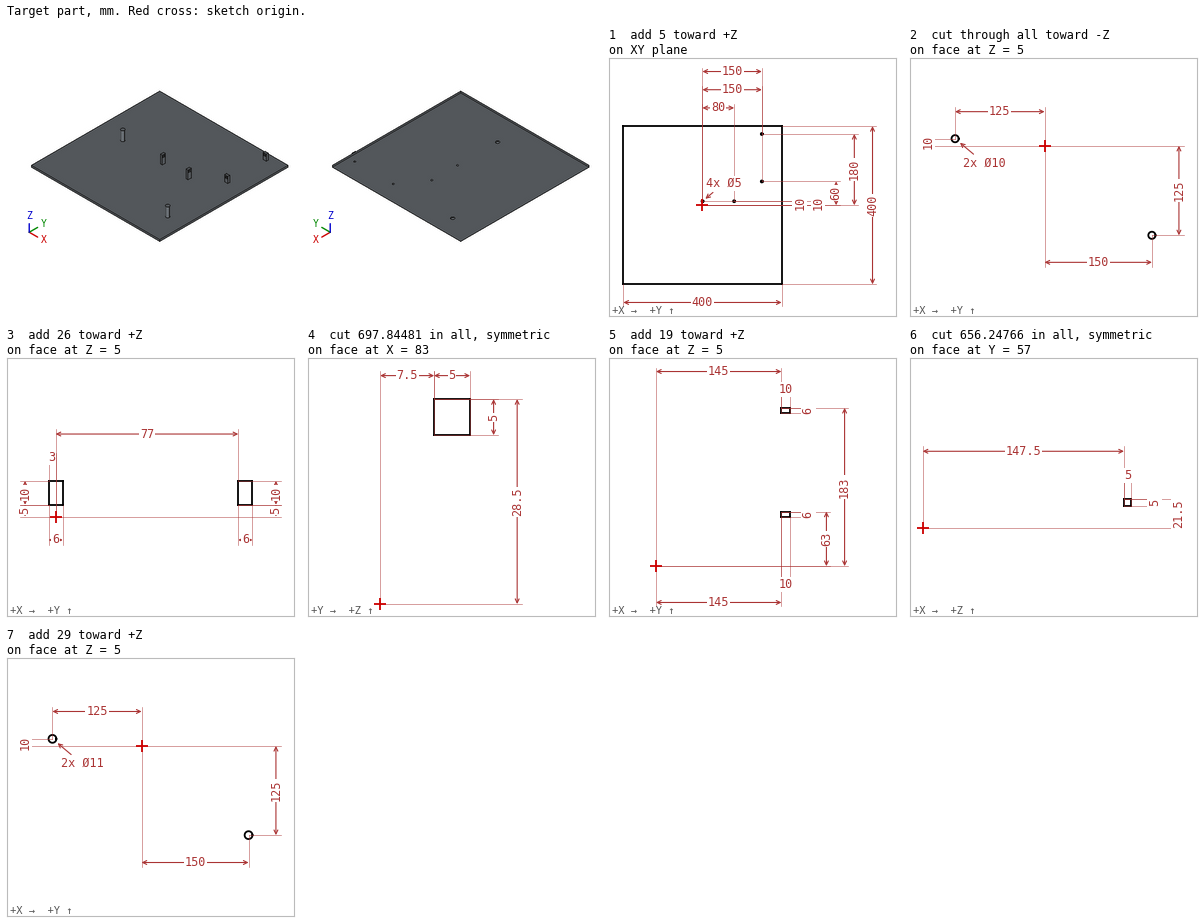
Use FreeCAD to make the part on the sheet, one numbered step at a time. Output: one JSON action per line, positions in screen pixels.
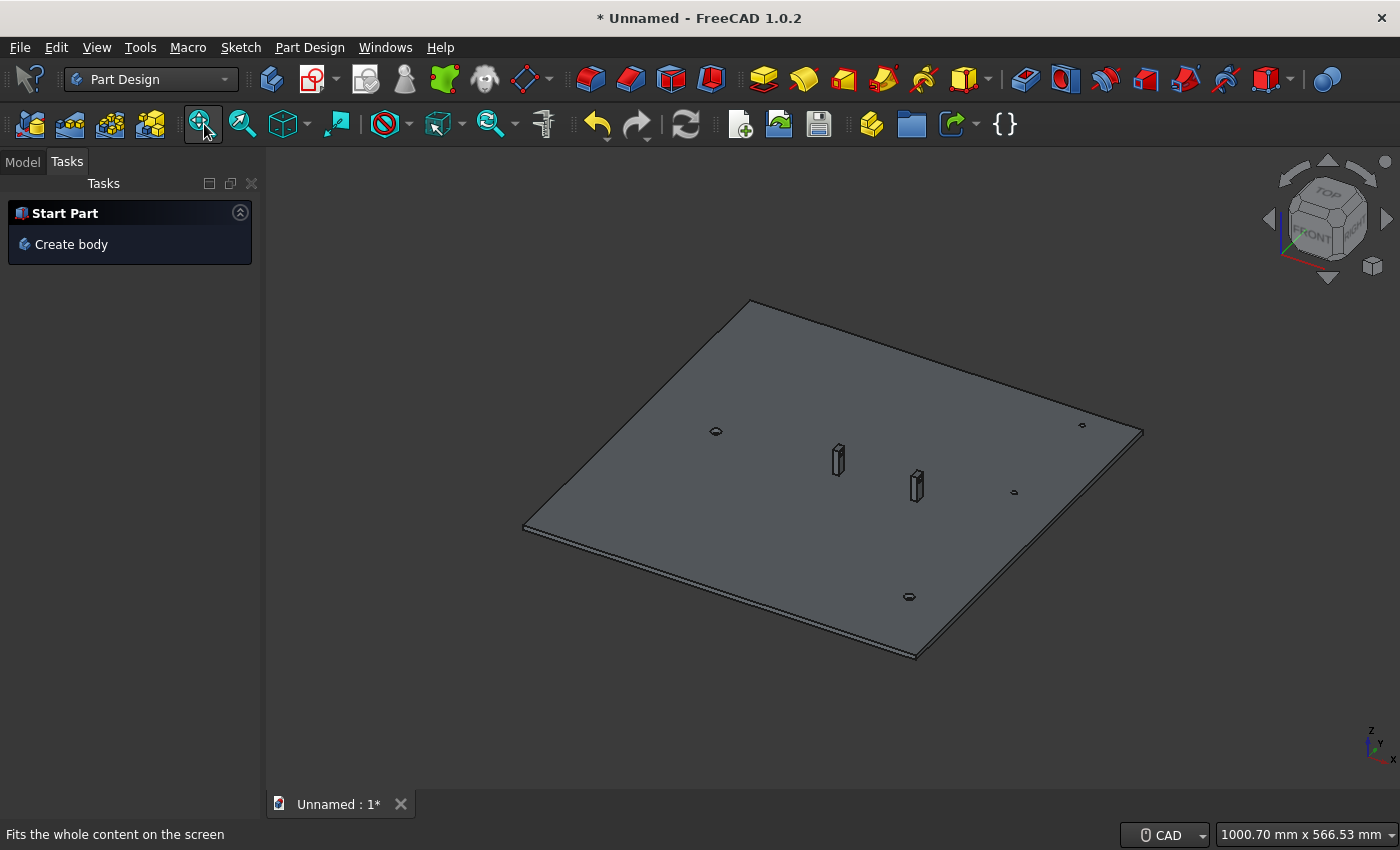
{"action": "left_click", "coordinate": [954, 431]}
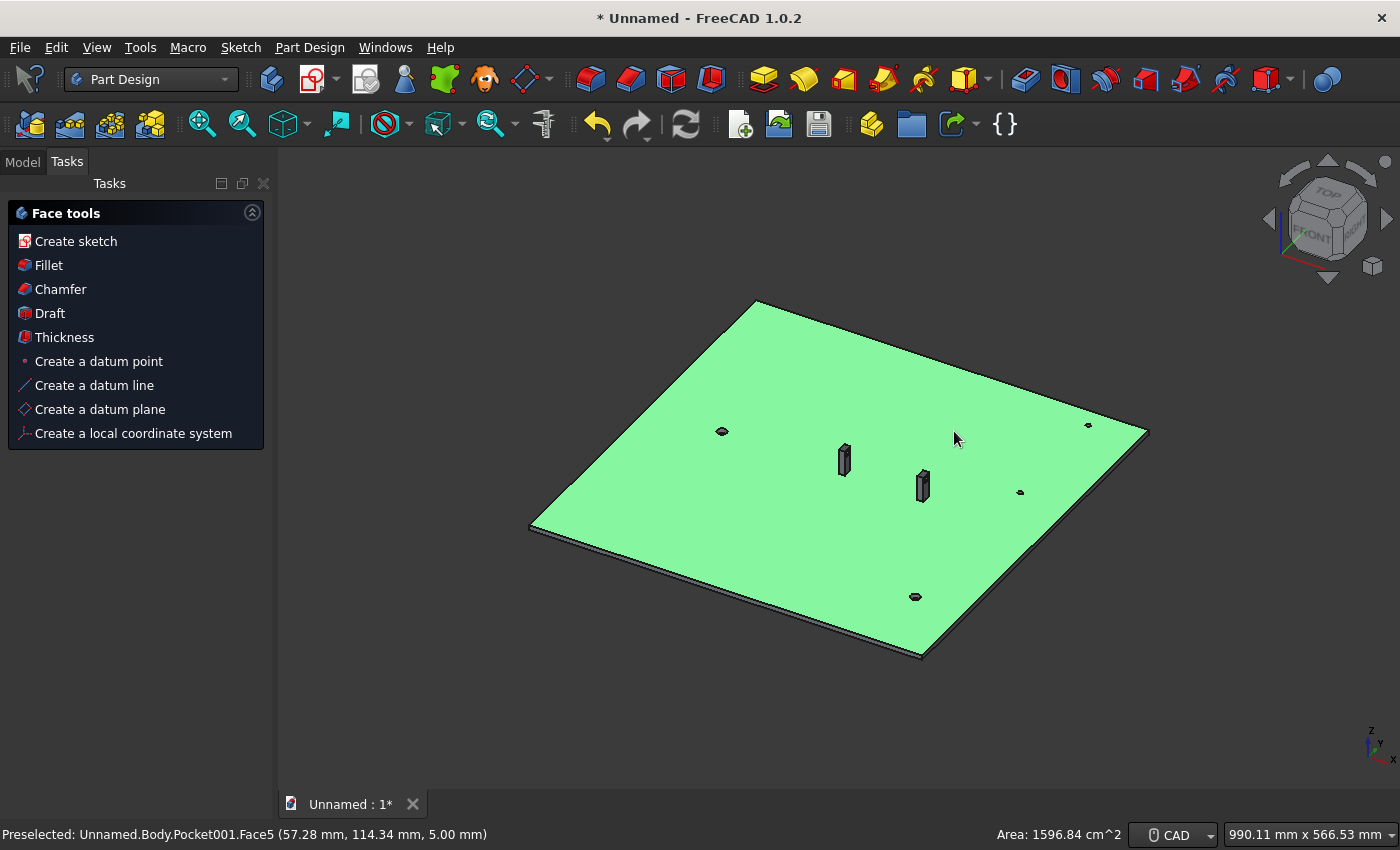
{"action": "left_click", "coordinate": [312, 80]}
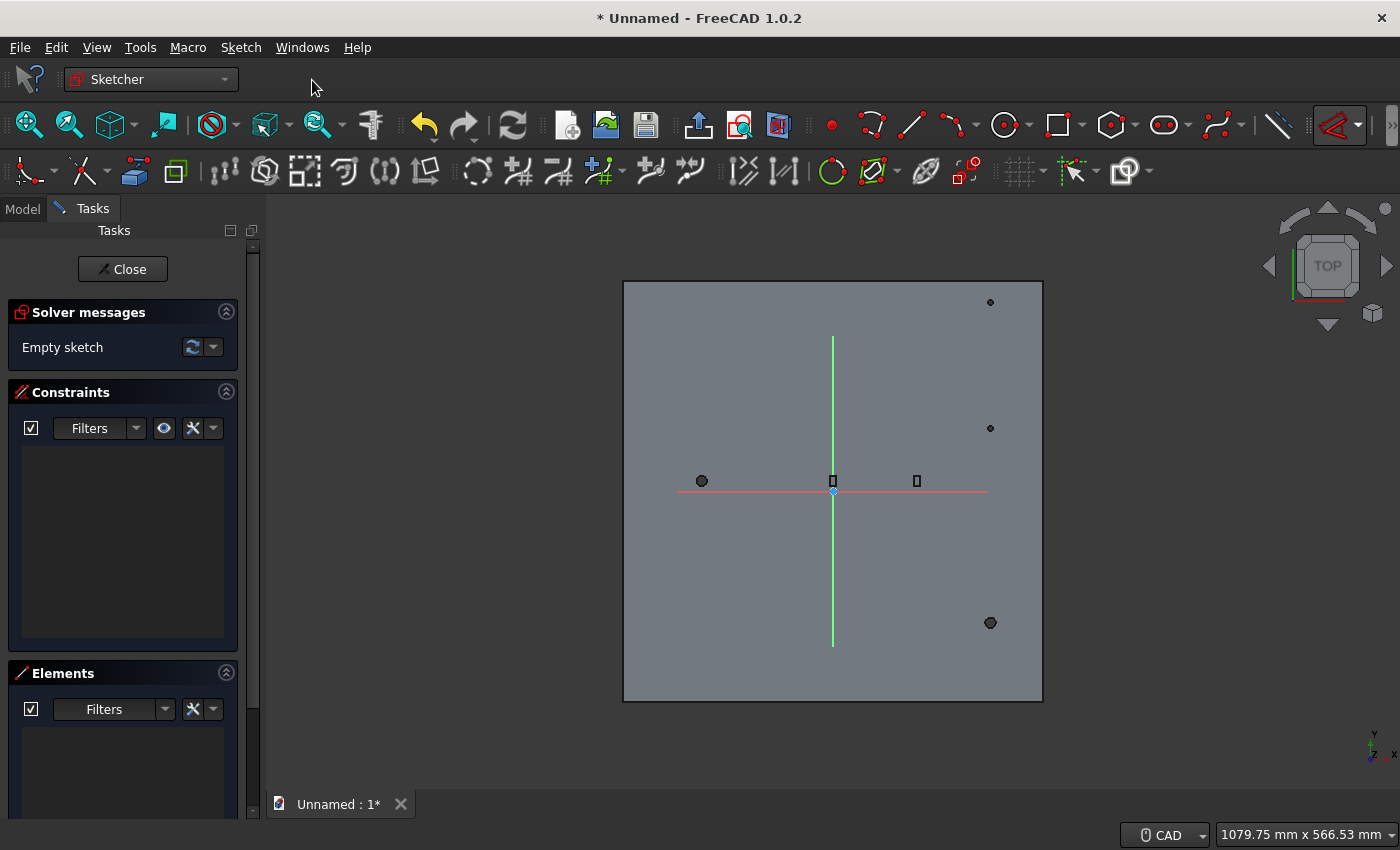
{"action": "key", "text": "q s"}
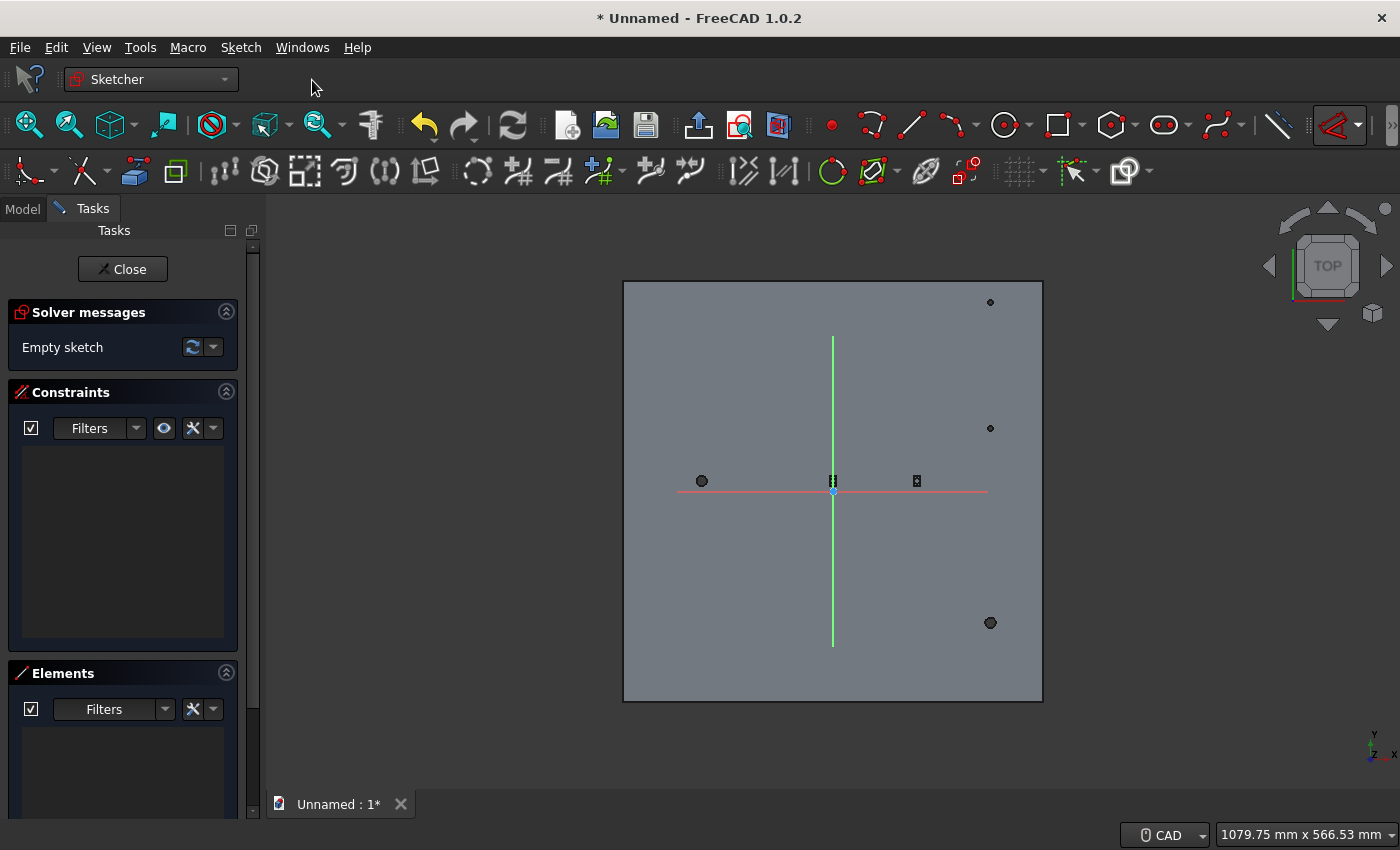
{"action": "scroll", "coordinate": [1097, 279], "scroll_direction": "up", "scroll_amount": 3}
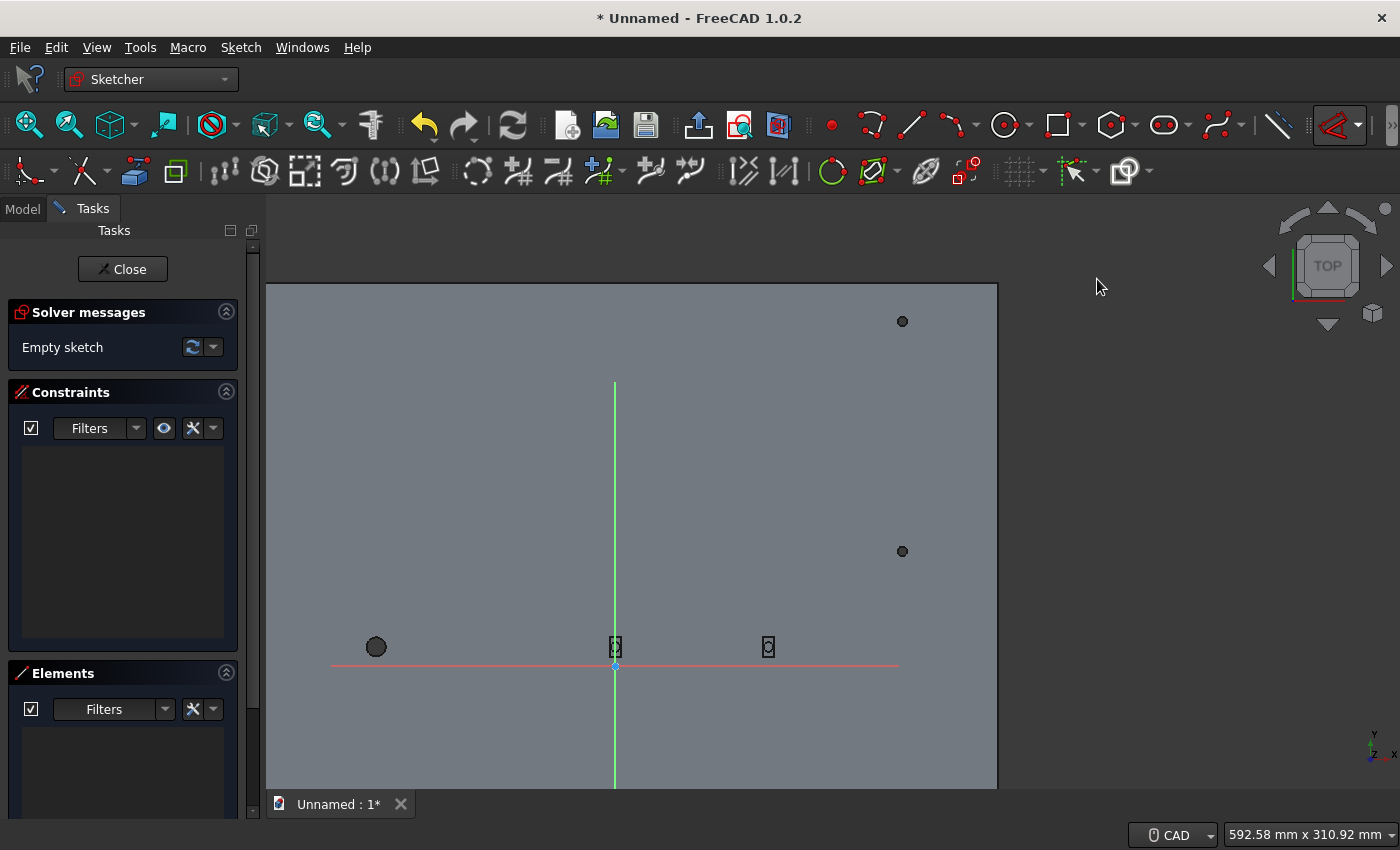
{"action": "key", "text": "g r"}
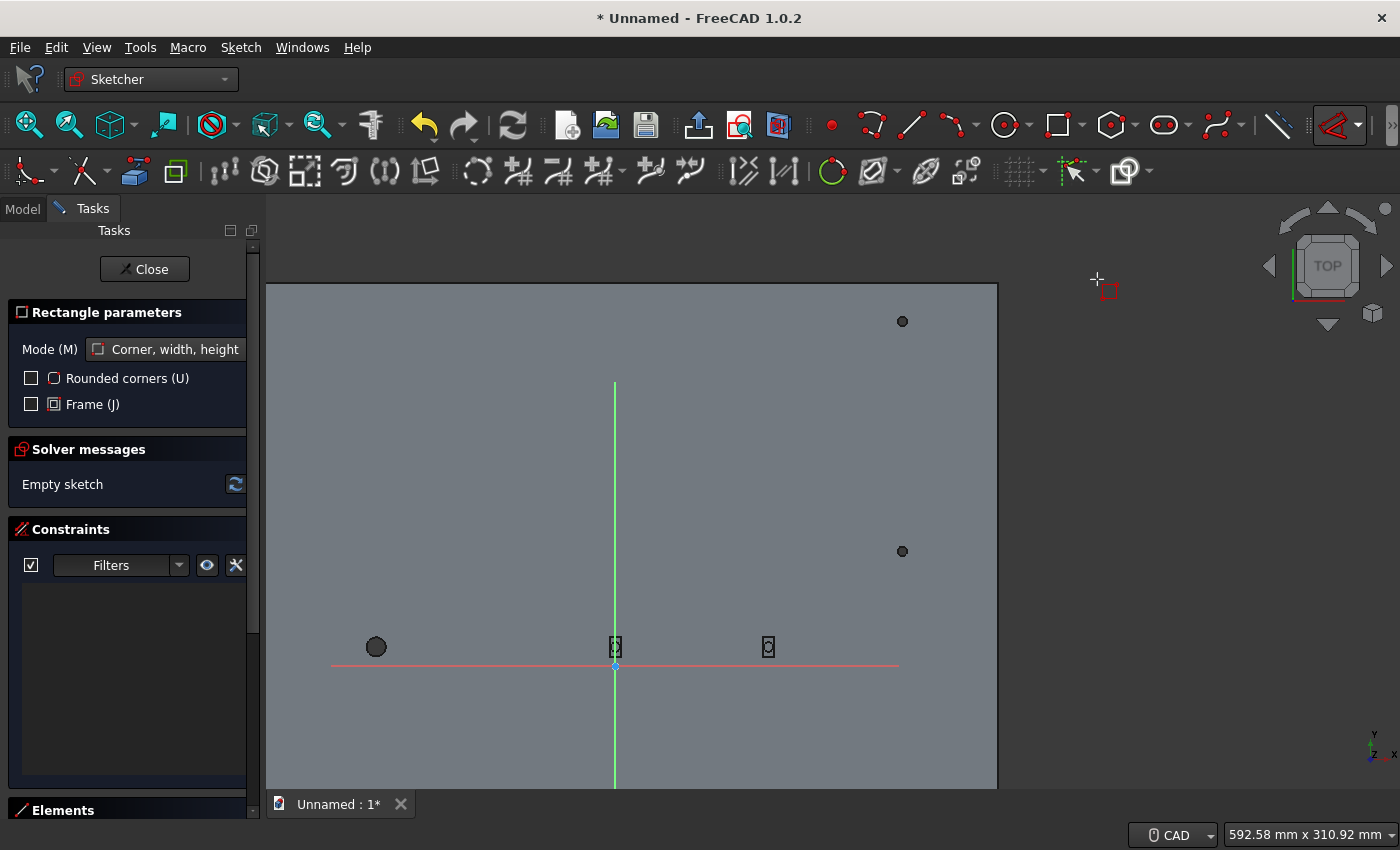
{"action": "scroll", "coordinate": [893, 316], "scroll_direction": "up", "scroll_amount": 2}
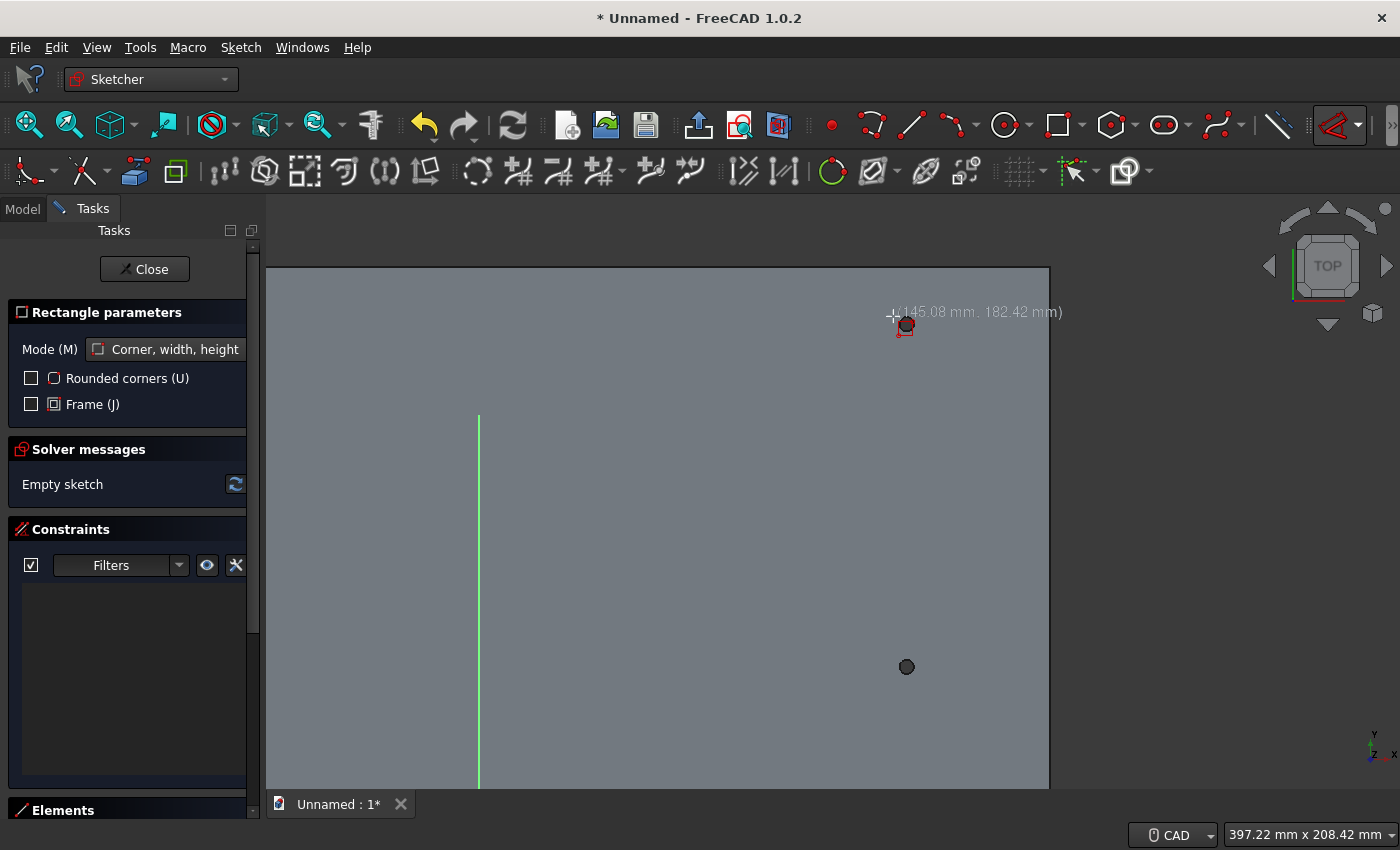
{"action": "left_click", "coordinate": [892, 316]}
{"action": "left_click", "coordinate": [921, 333]}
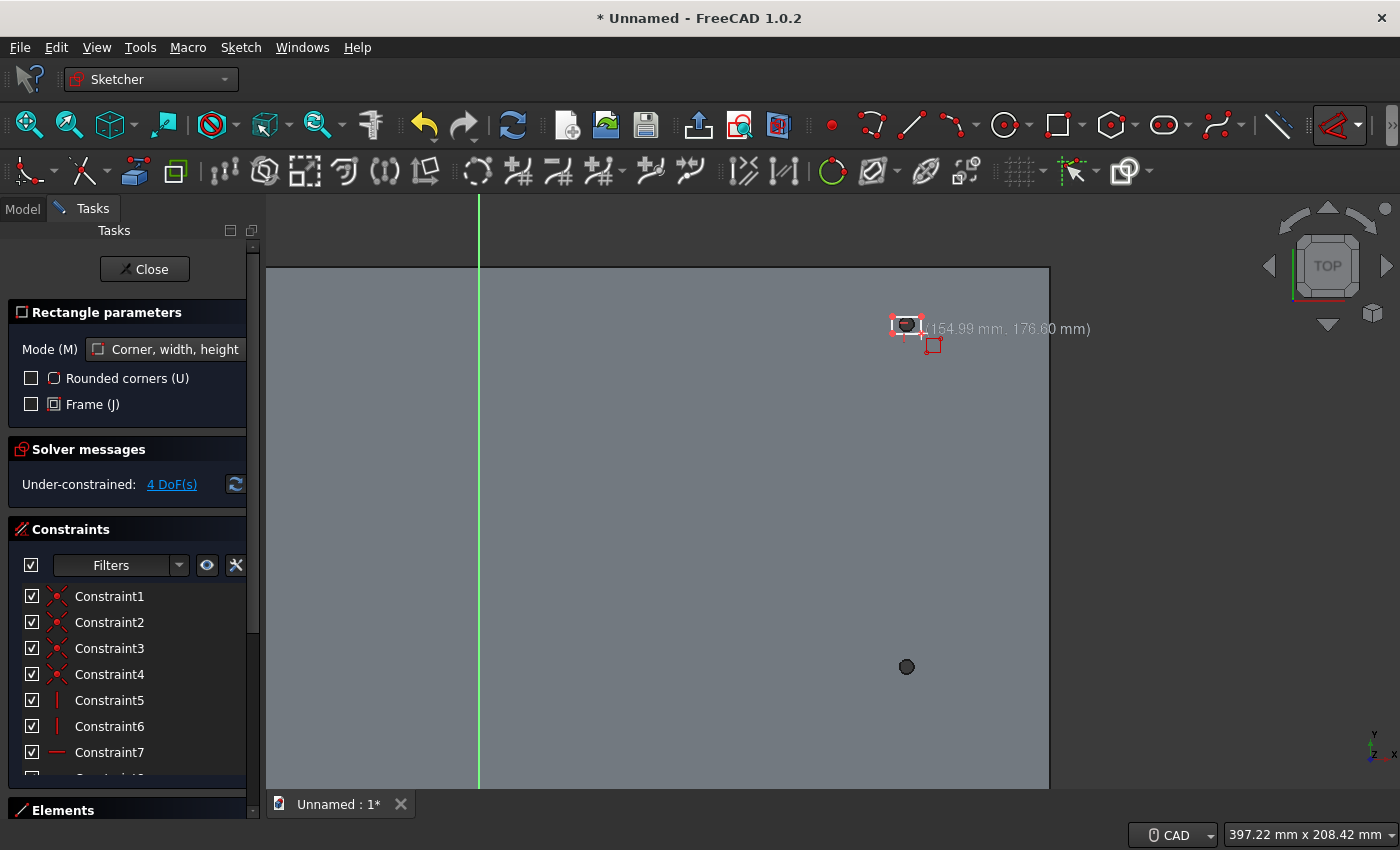
{"action": "left_click", "coordinate": [892, 658]}
{"action": "left_click", "coordinate": [921, 675]}
{"action": "key", "text": "Escape"}